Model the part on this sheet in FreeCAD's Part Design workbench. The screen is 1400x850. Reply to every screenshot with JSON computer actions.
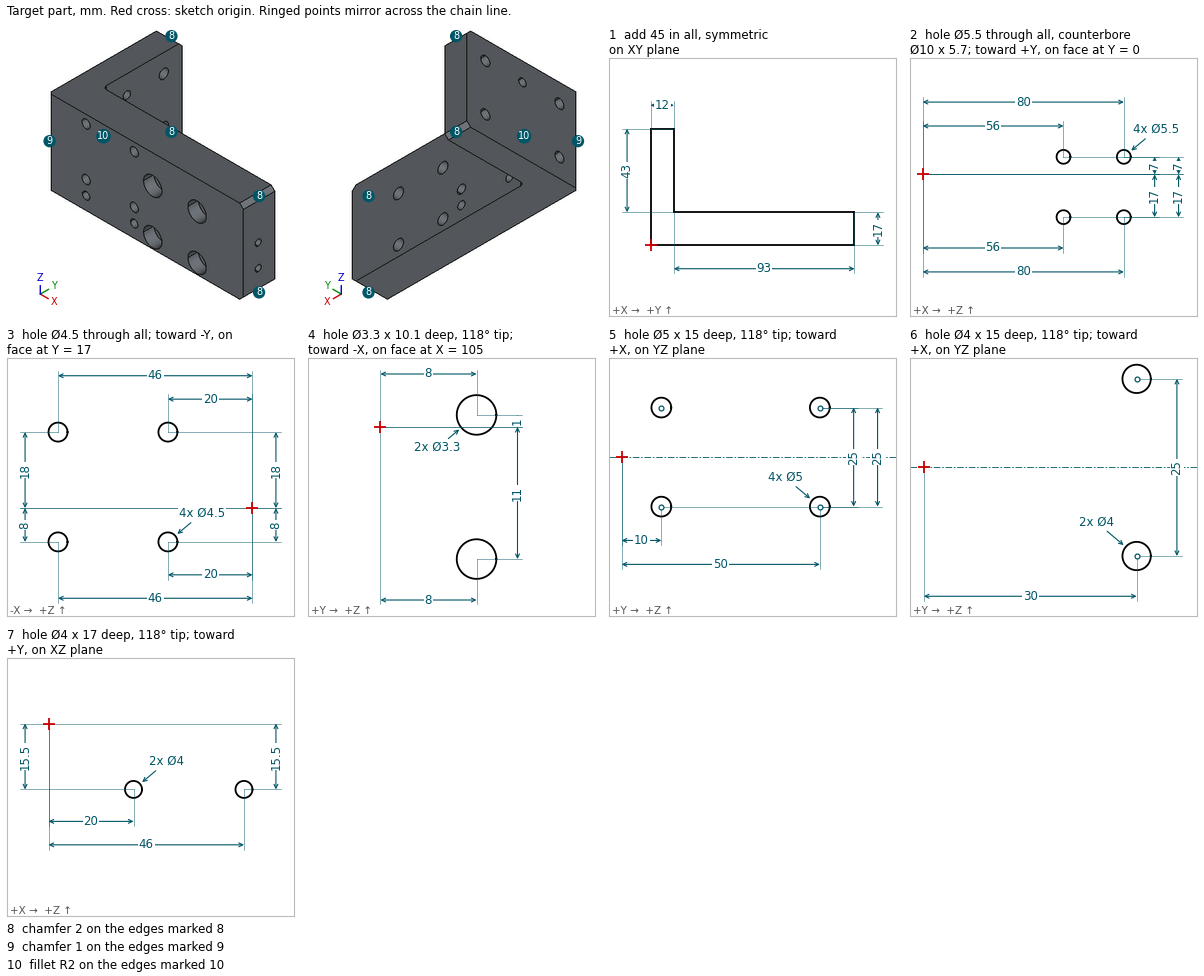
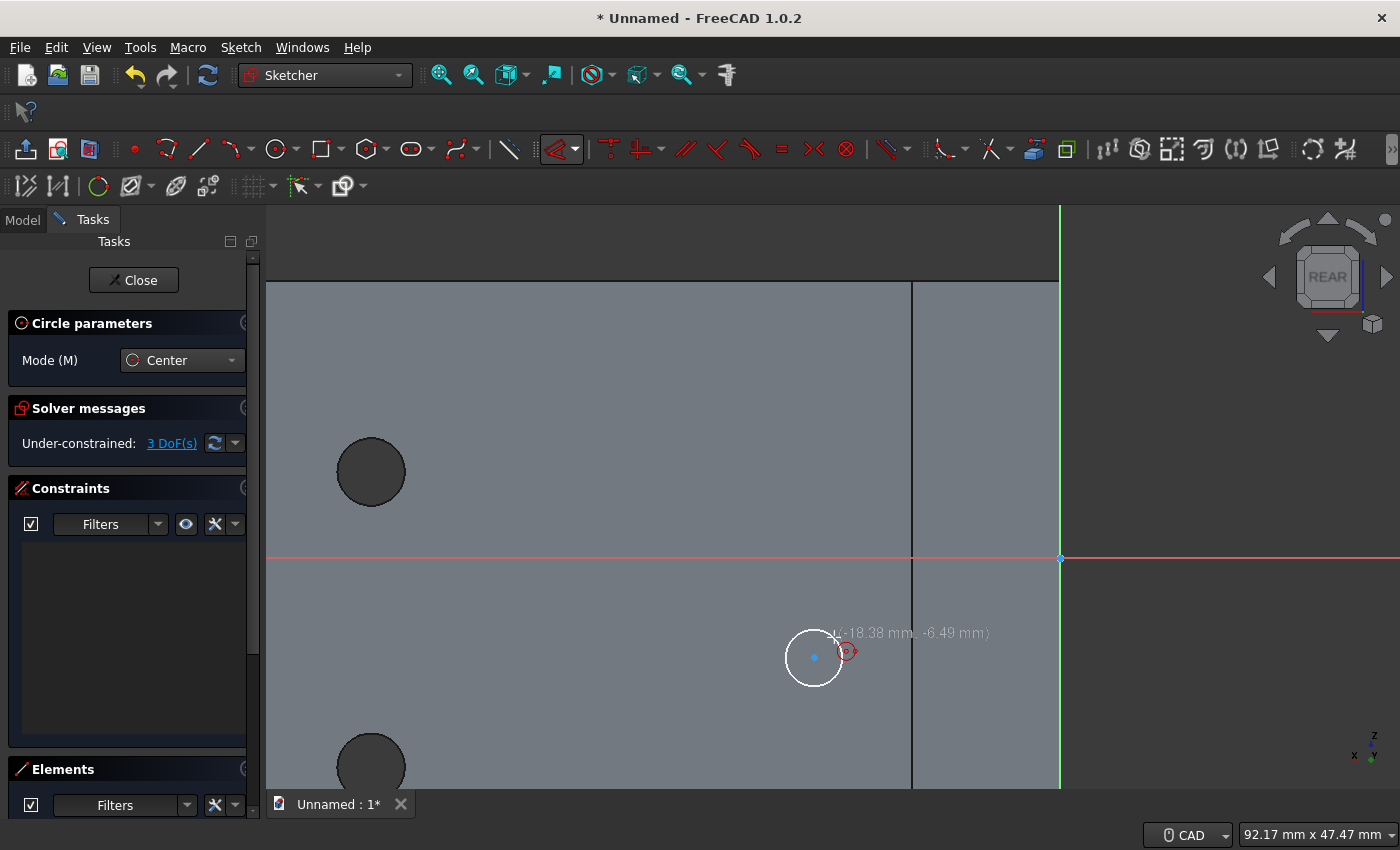
{"action": "left_click", "coordinate": [494, 657]}
{"action": "left_click", "coordinate": [514, 637]}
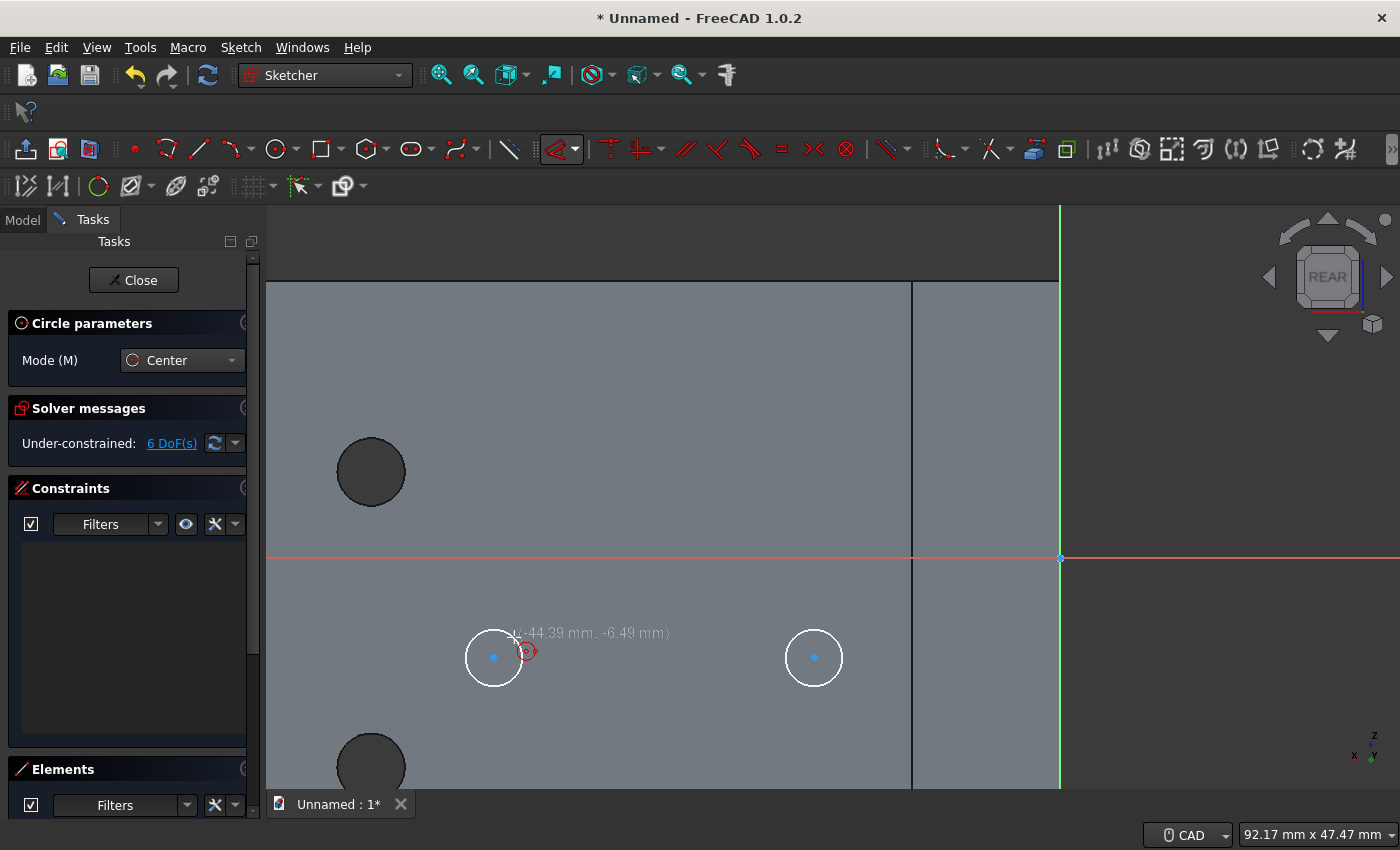
{"action": "left_click", "coordinate": [814, 337]}
{"action": "left_click", "coordinate": [834, 317]}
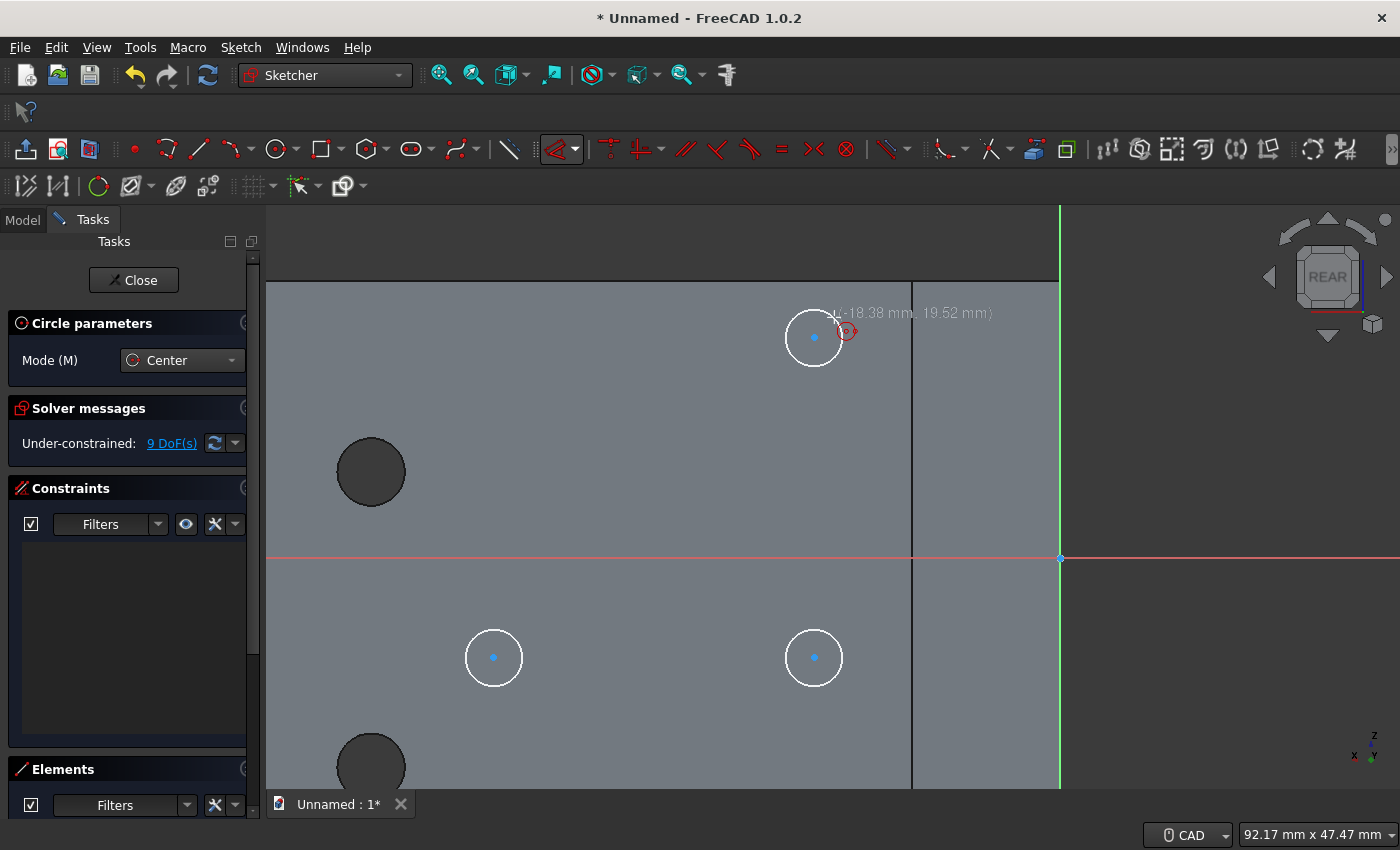
{"action": "left_click", "coordinate": [494, 337]}
{"action": "left_click", "coordinate": [514, 317]}
{"action": "key", "text": "Escape"}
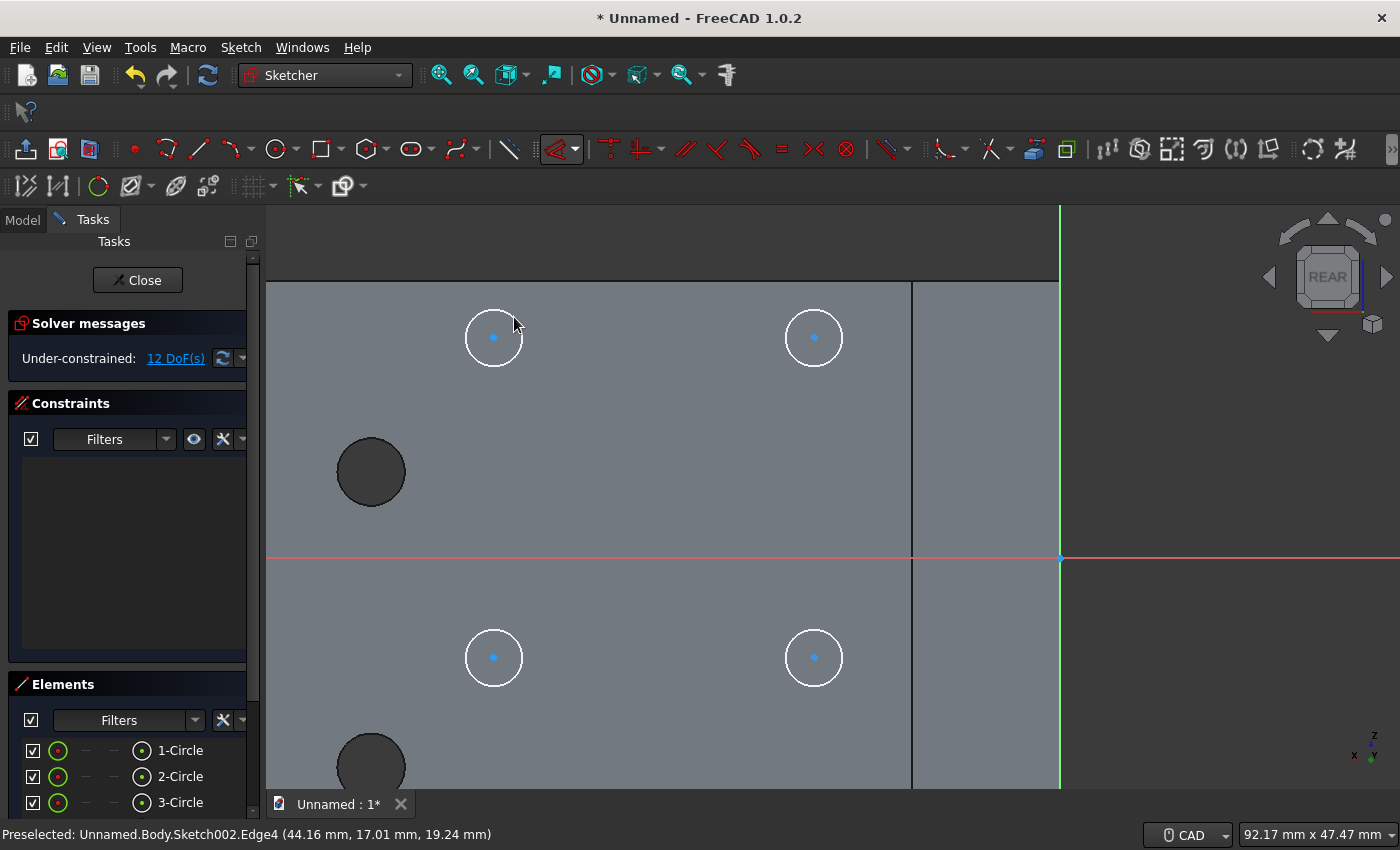
{"action": "left_click", "coordinate": [834, 638]}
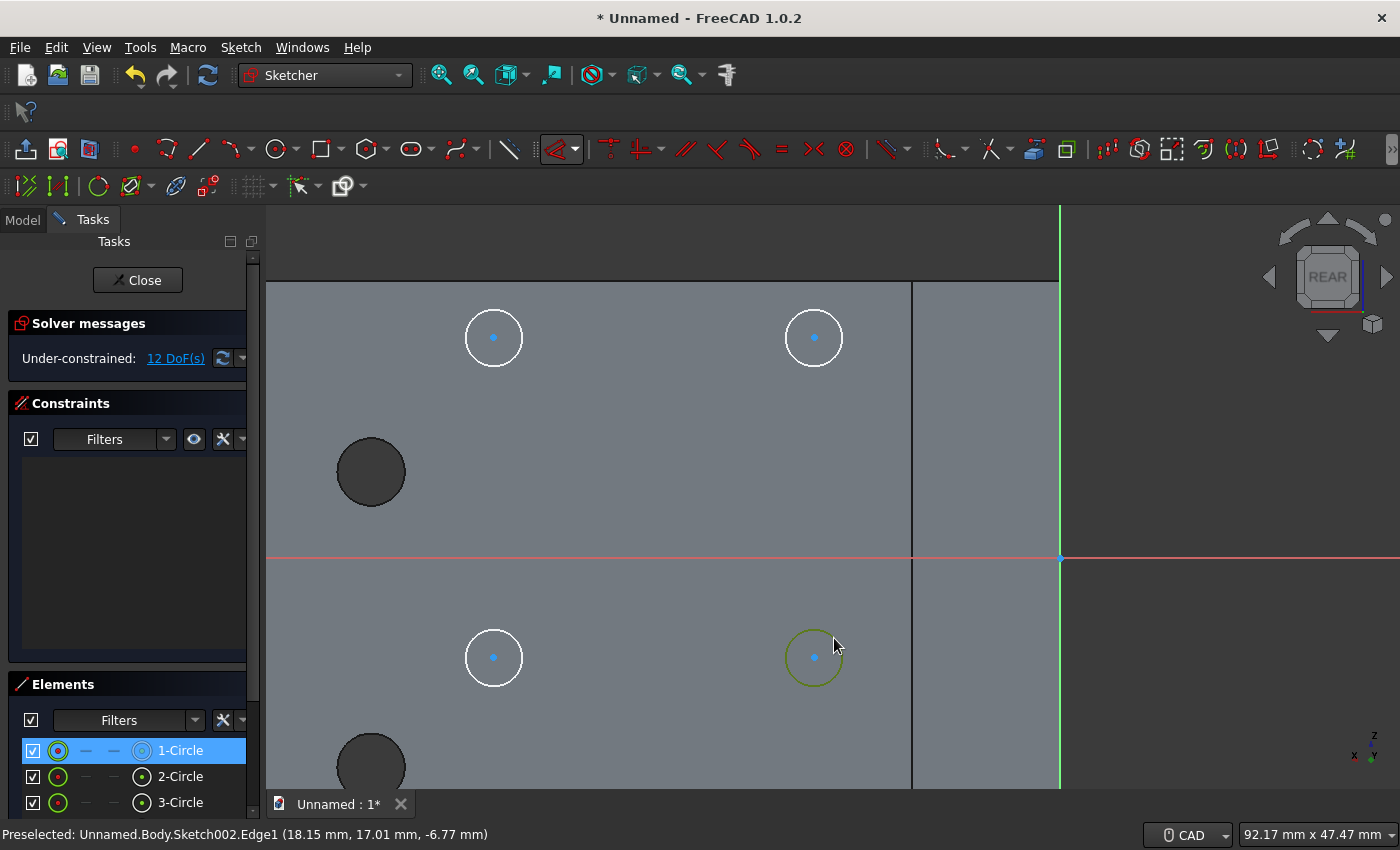
{"action": "left_click", "coordinate": [514, 638]}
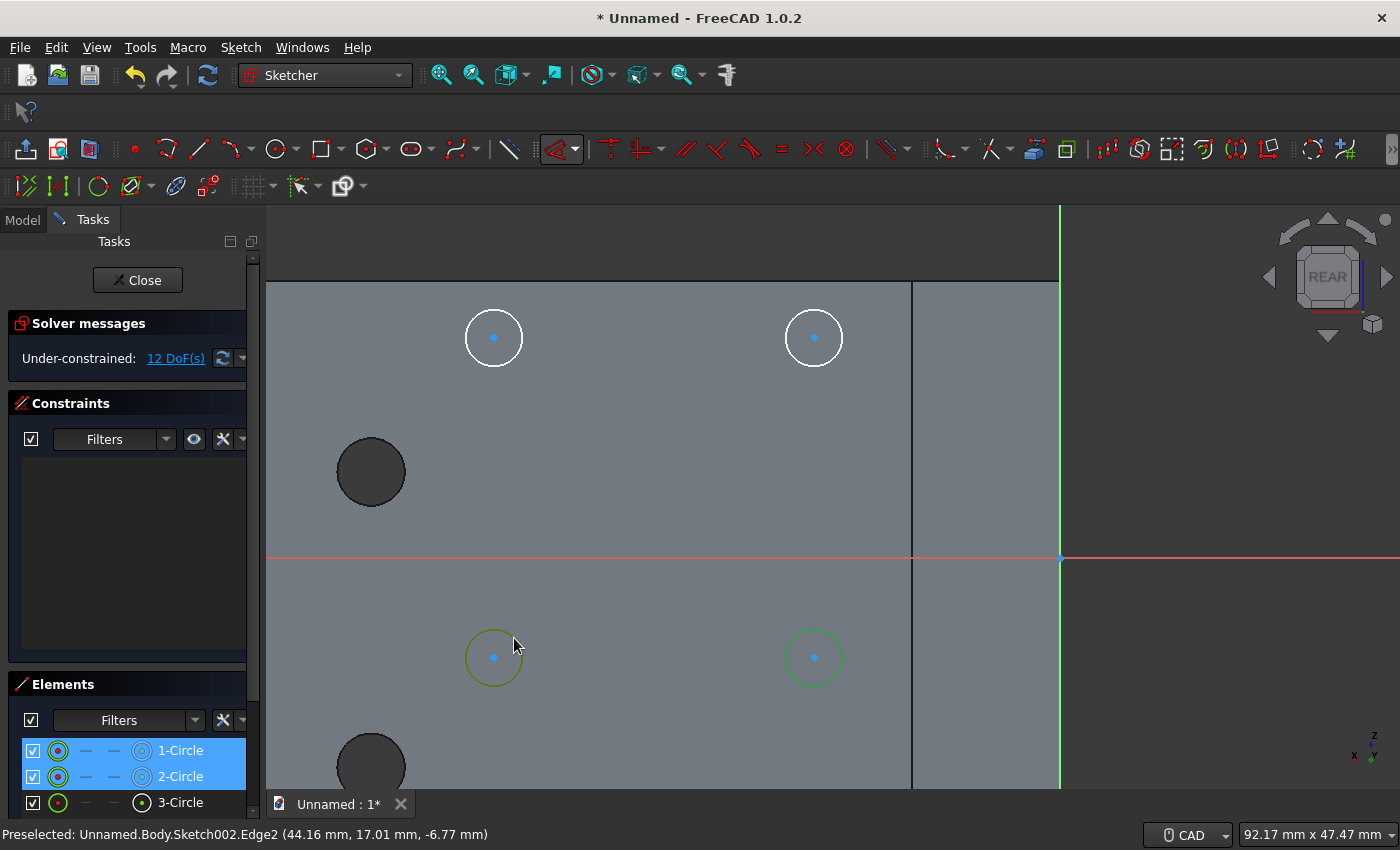
{"action": "left_click", "coordinate": [834, 318]}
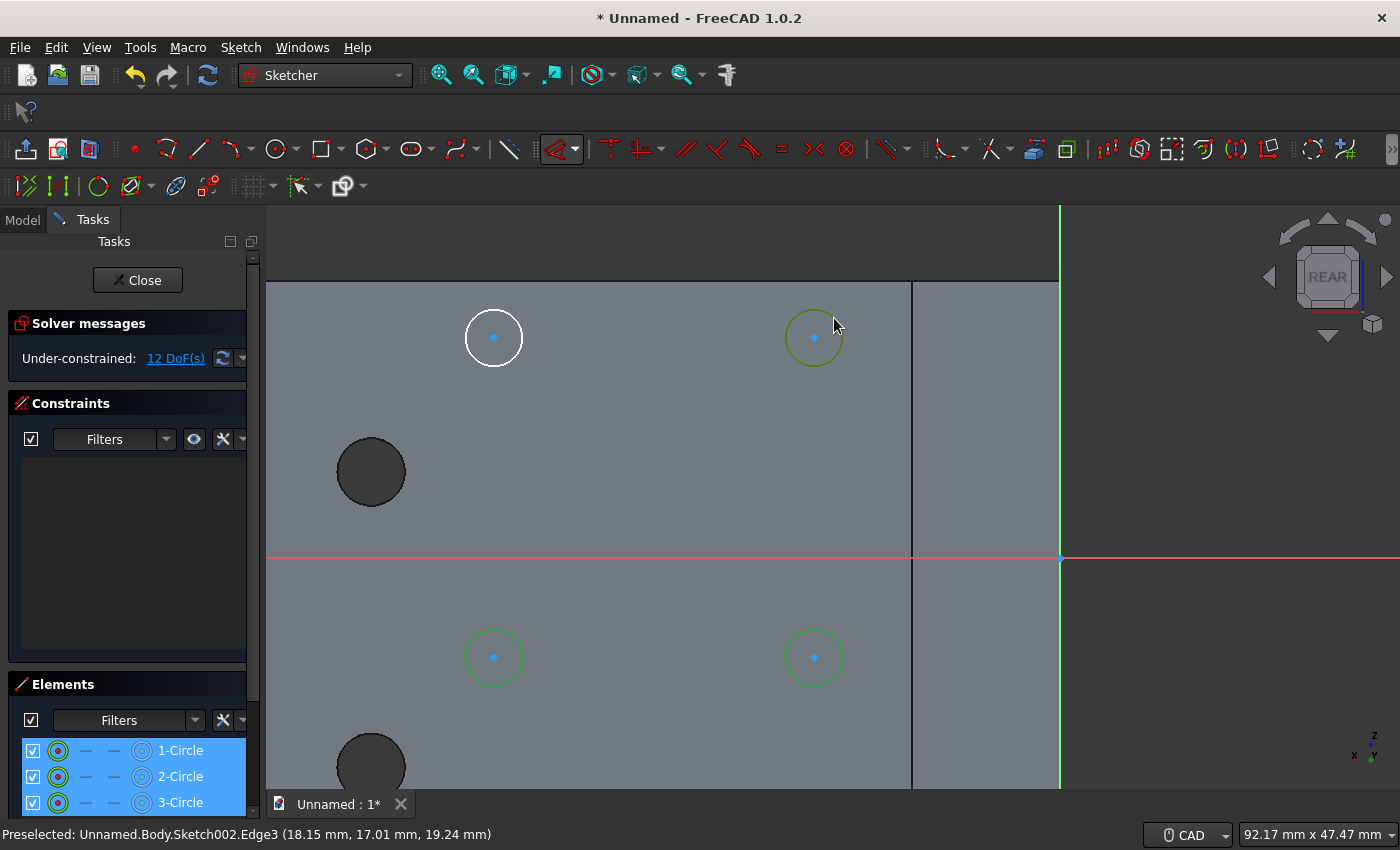
{"action": "left_click", "coordinate": [514, 318]}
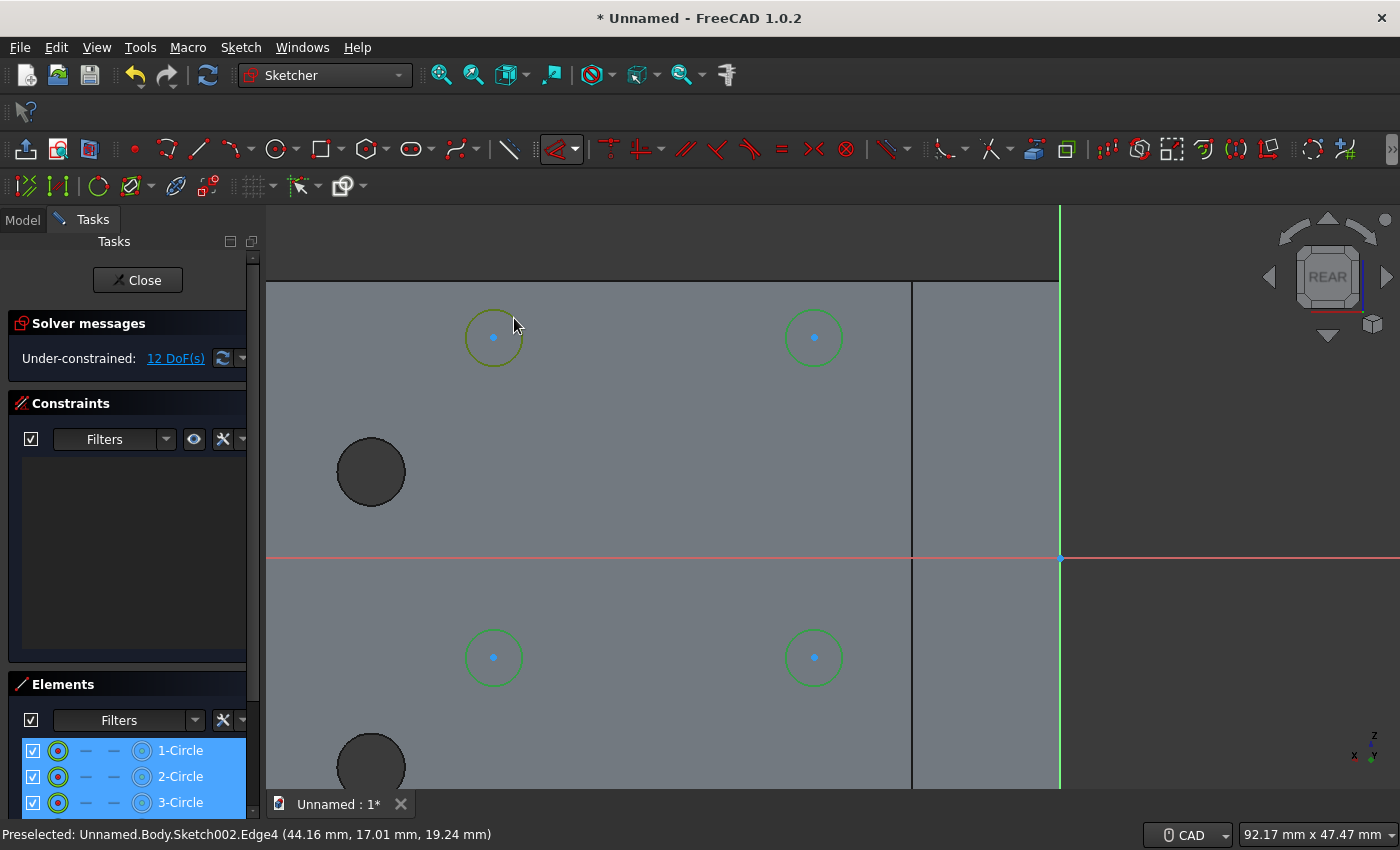
{"action": "key", "text": "e"}